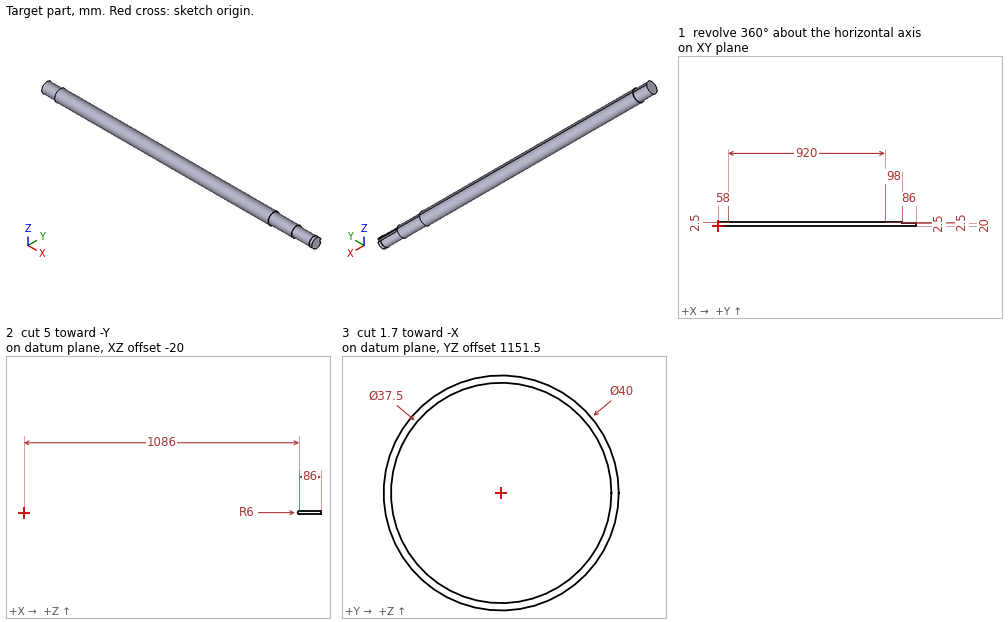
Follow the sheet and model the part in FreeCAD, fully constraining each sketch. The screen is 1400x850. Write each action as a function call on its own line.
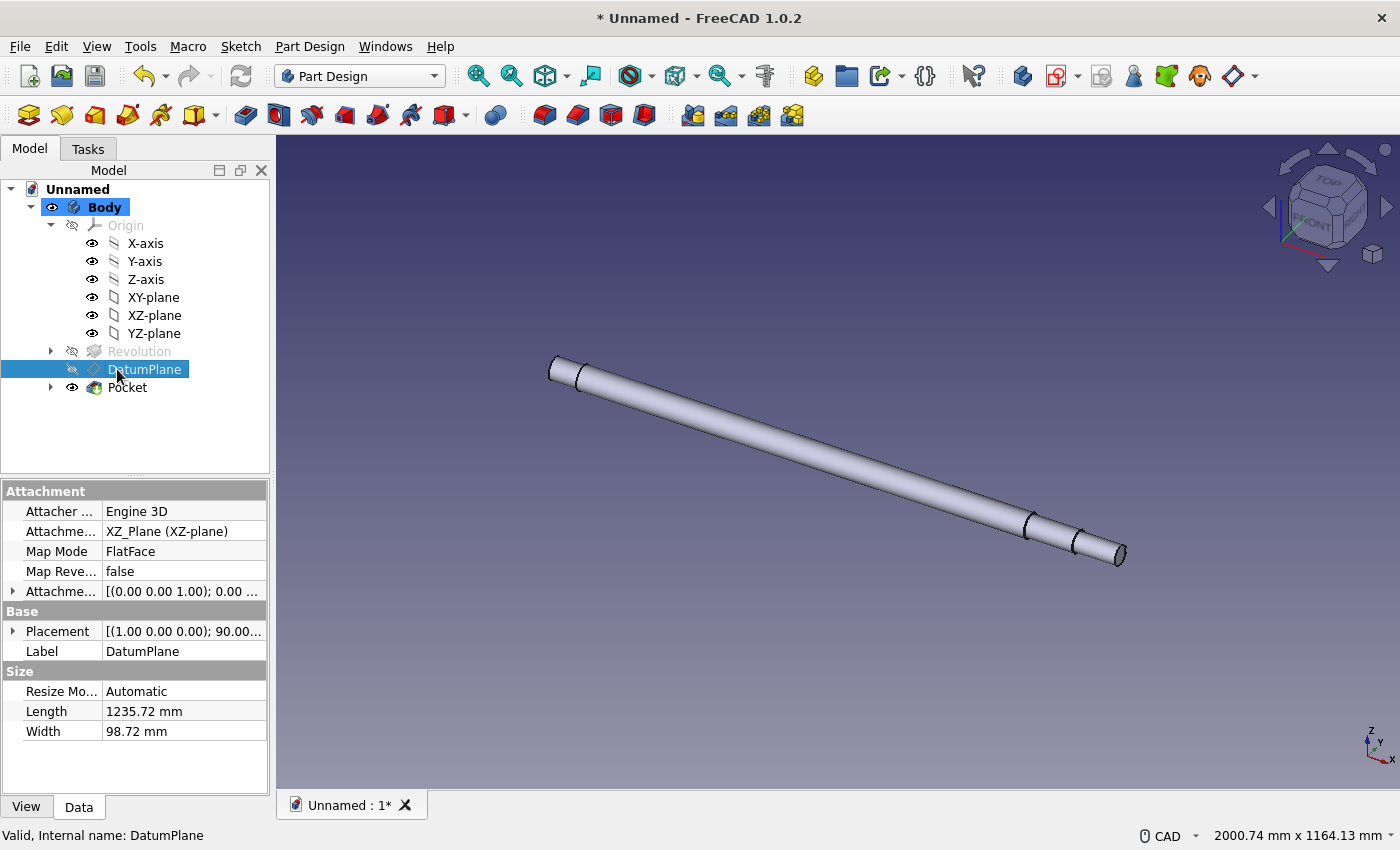
click(137, 333)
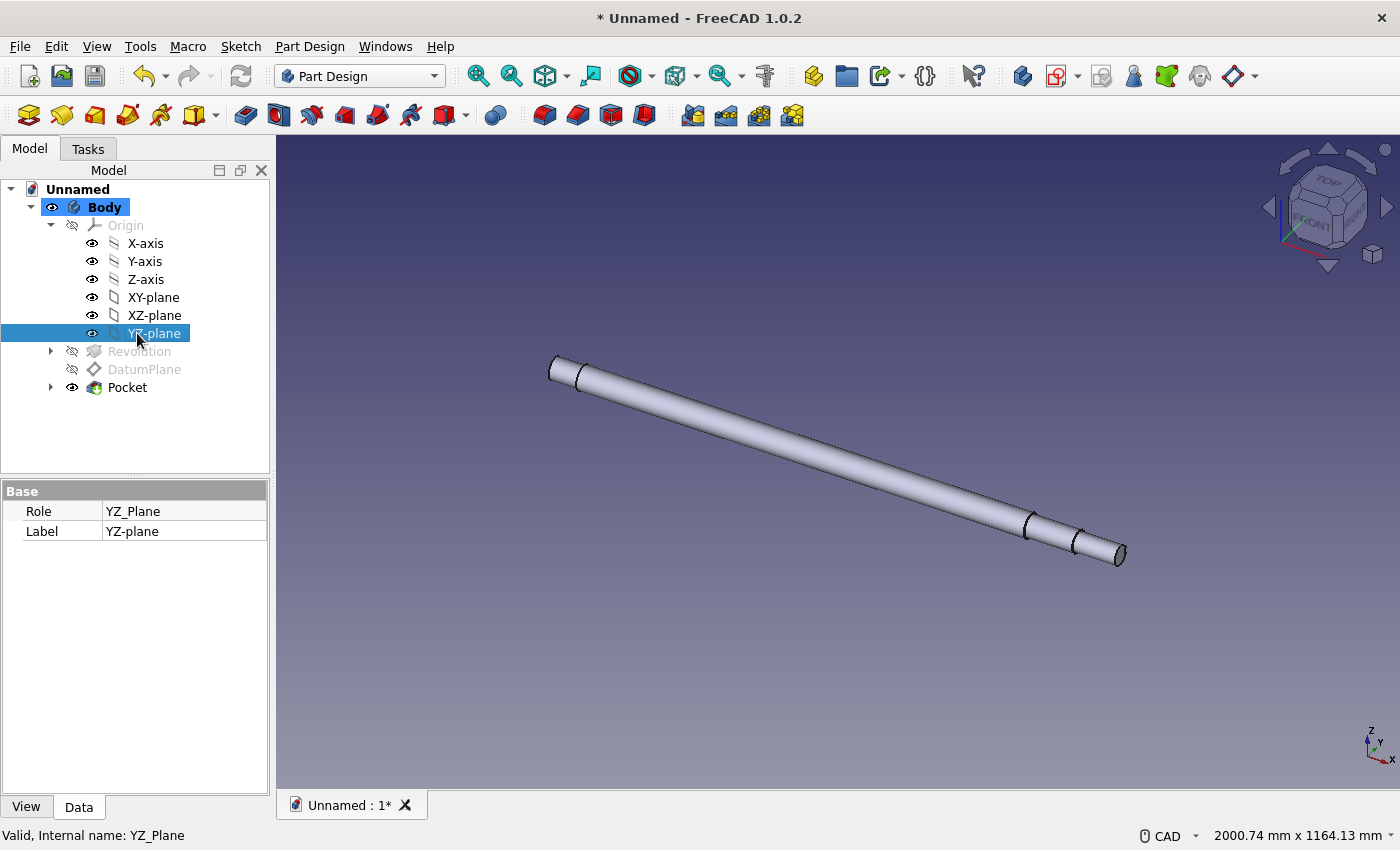
click(1232, 76)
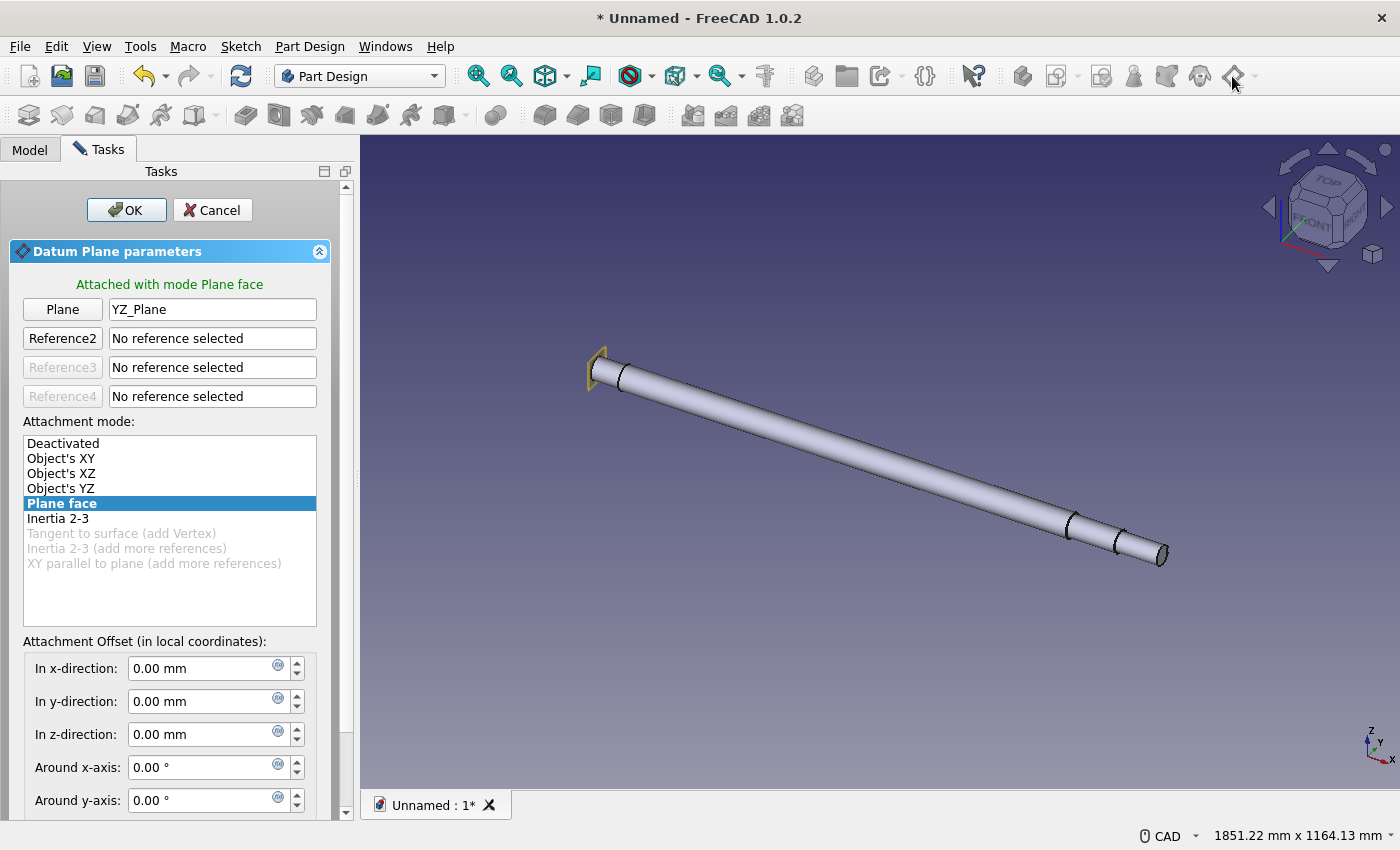
triple_click(210, 734)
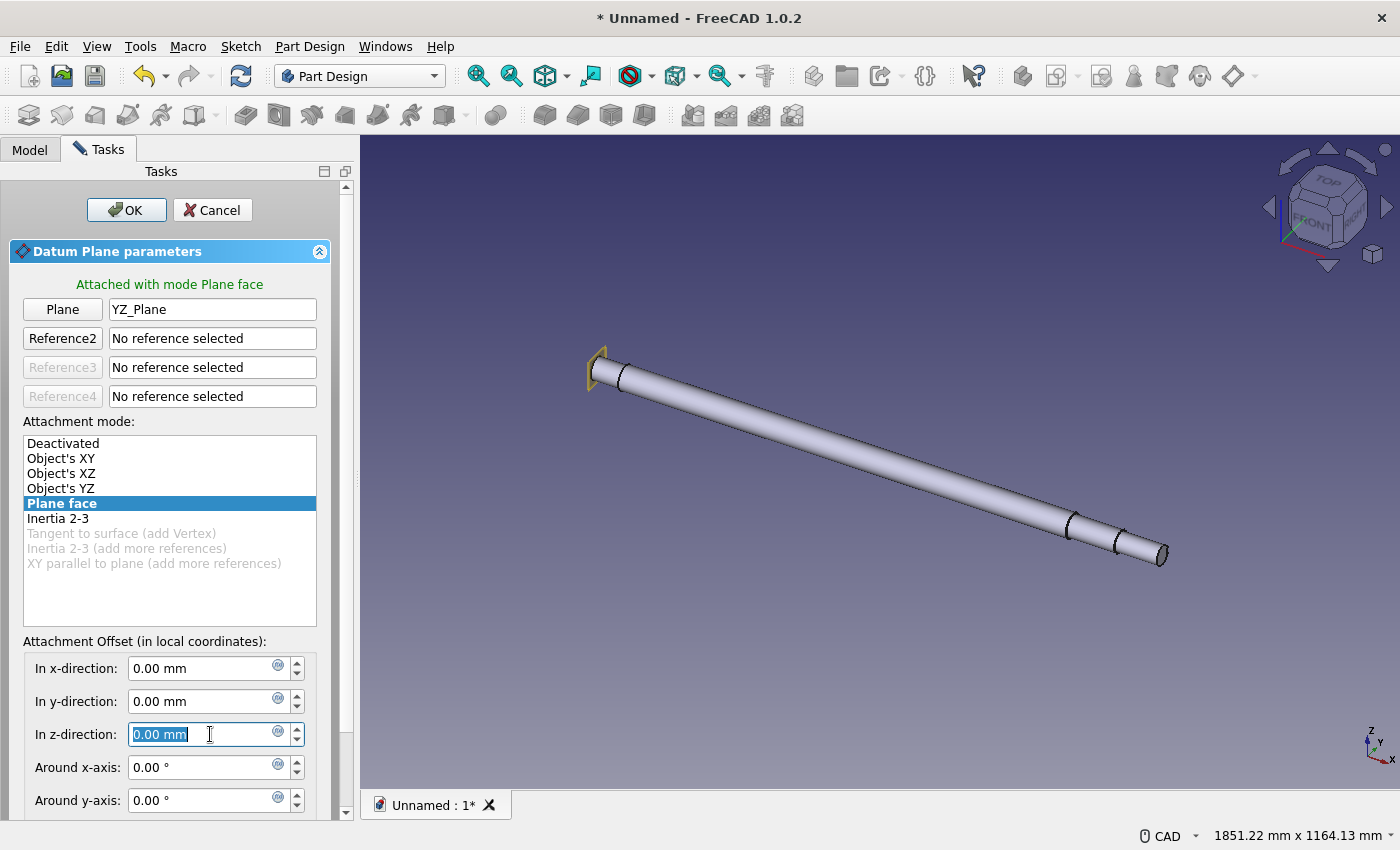
text(1151.5)
key(Tab)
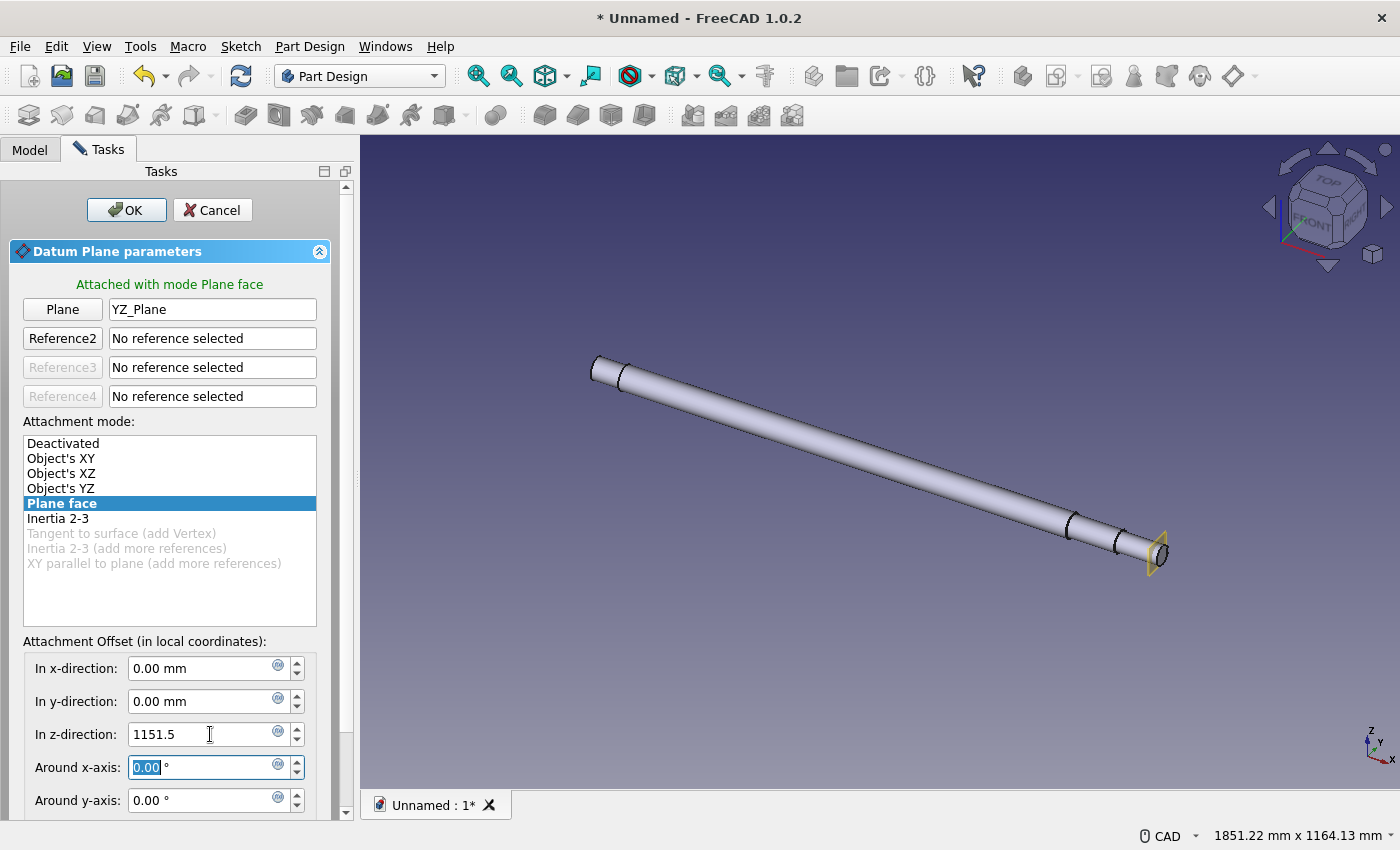
click(127, 210)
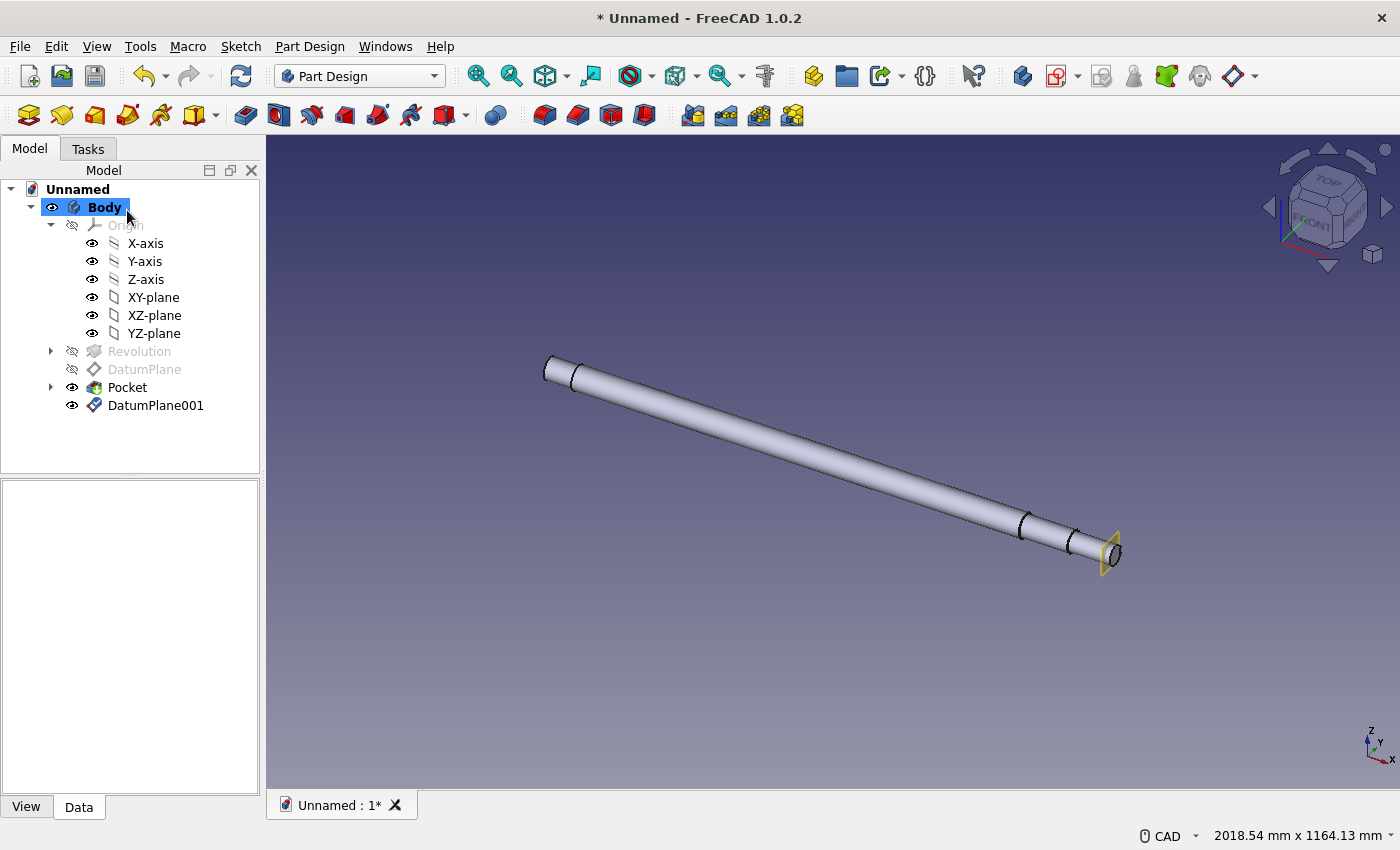
click(117, 405)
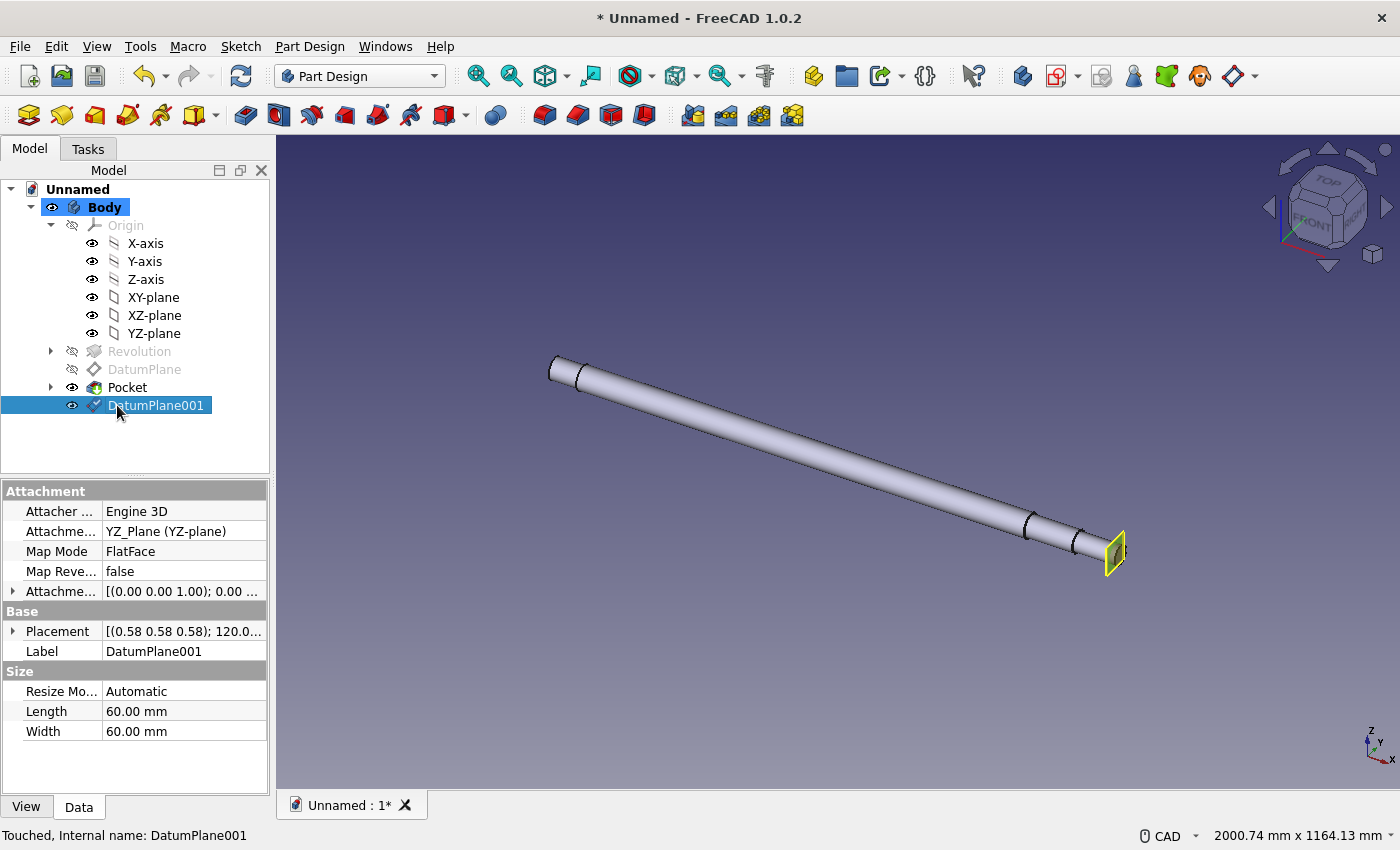
click(1056, 76)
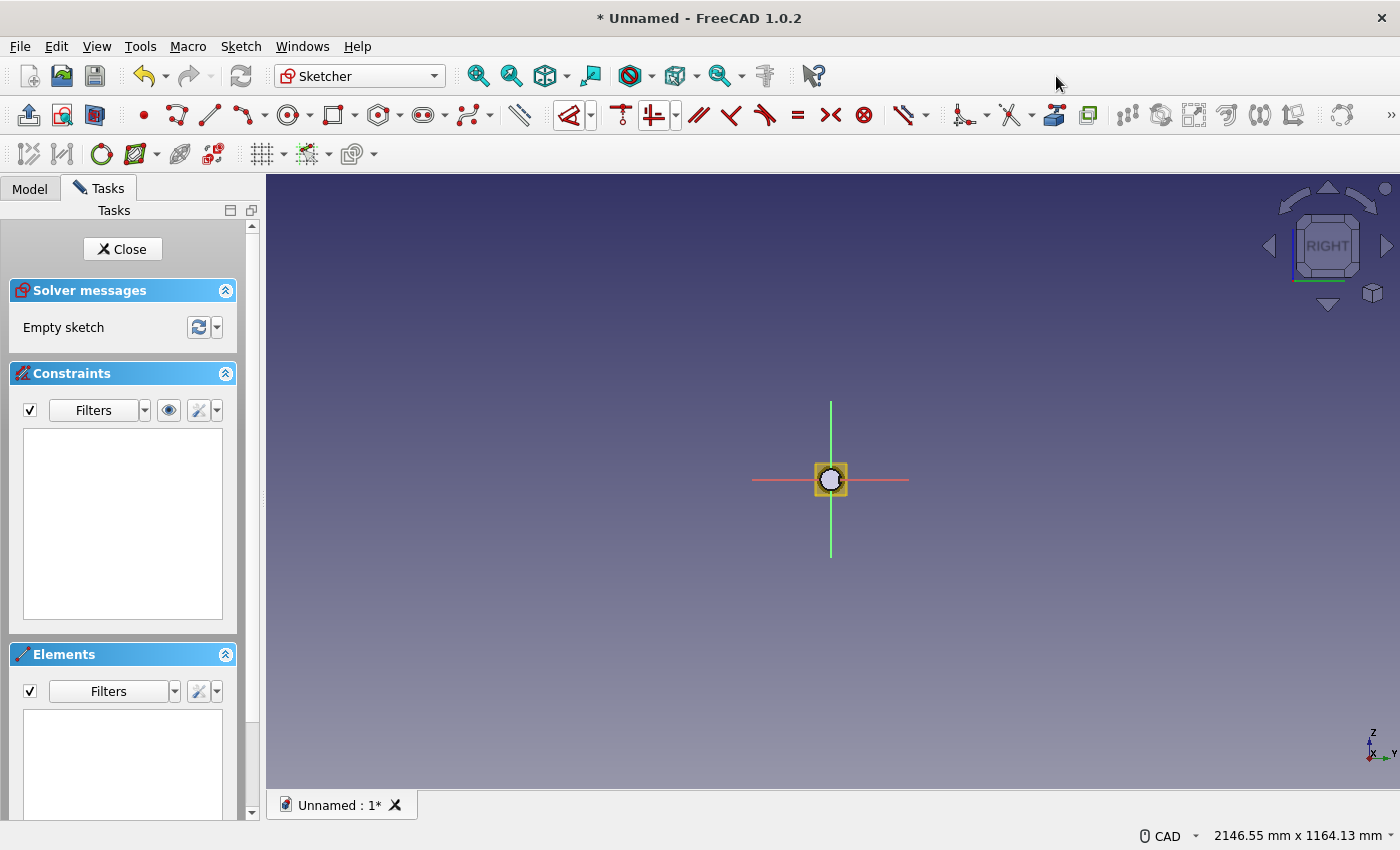
click(95, 116)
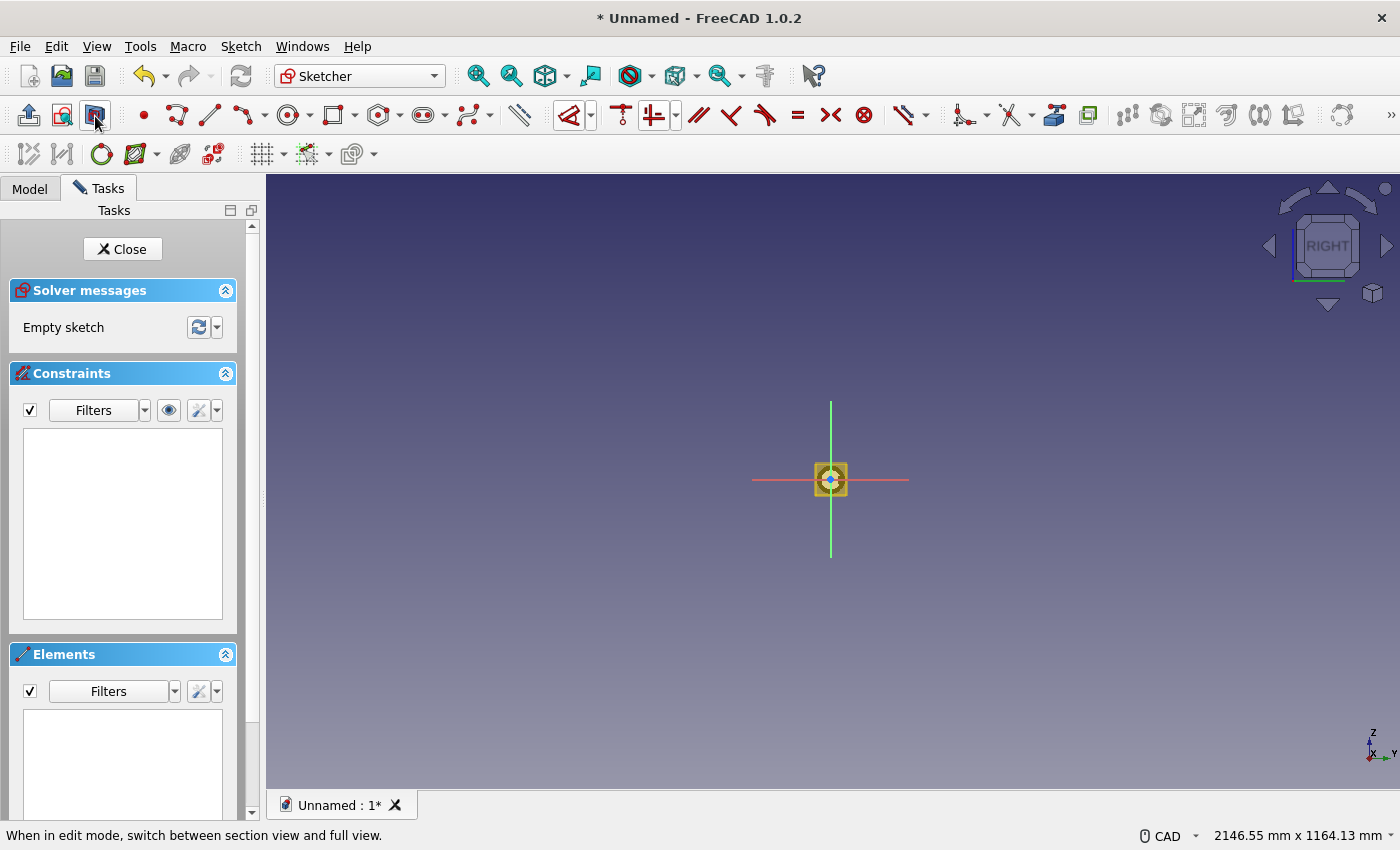
scroll(834, 480, up, 15)